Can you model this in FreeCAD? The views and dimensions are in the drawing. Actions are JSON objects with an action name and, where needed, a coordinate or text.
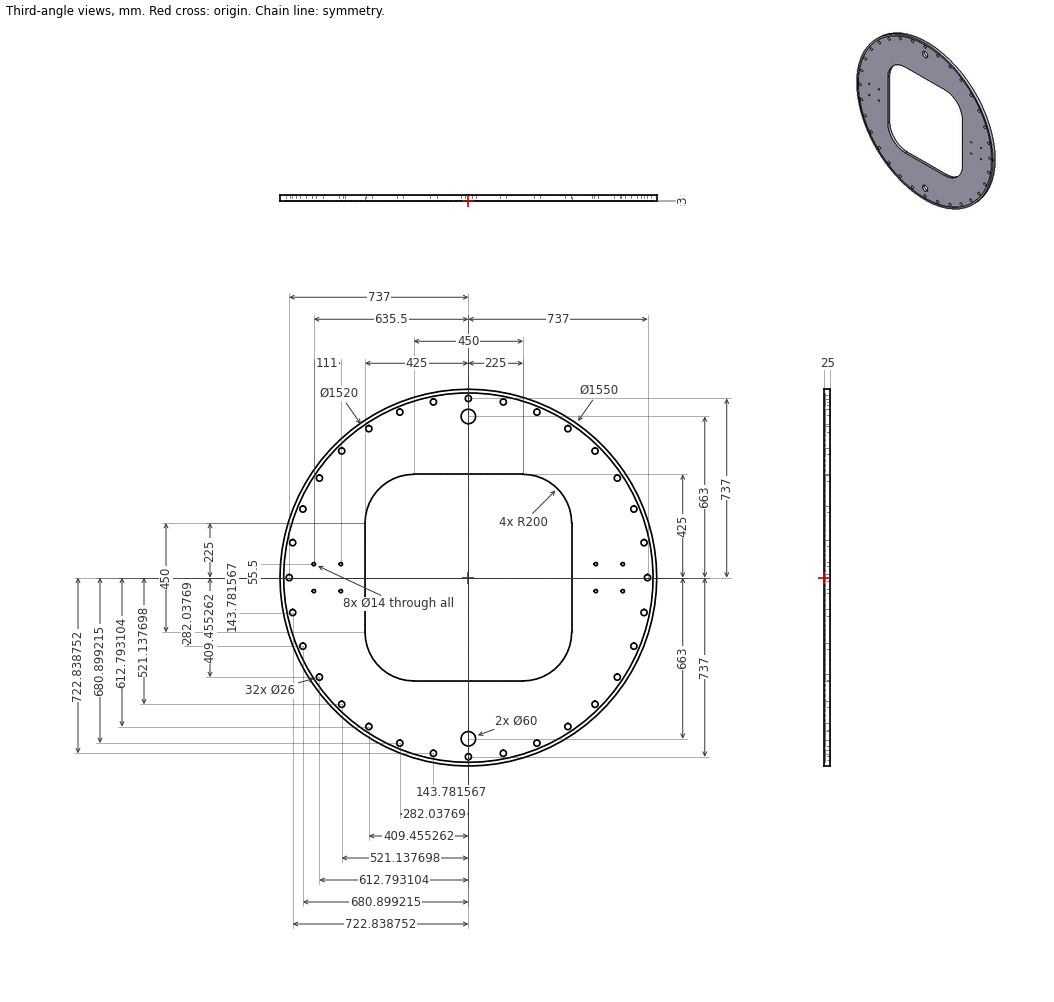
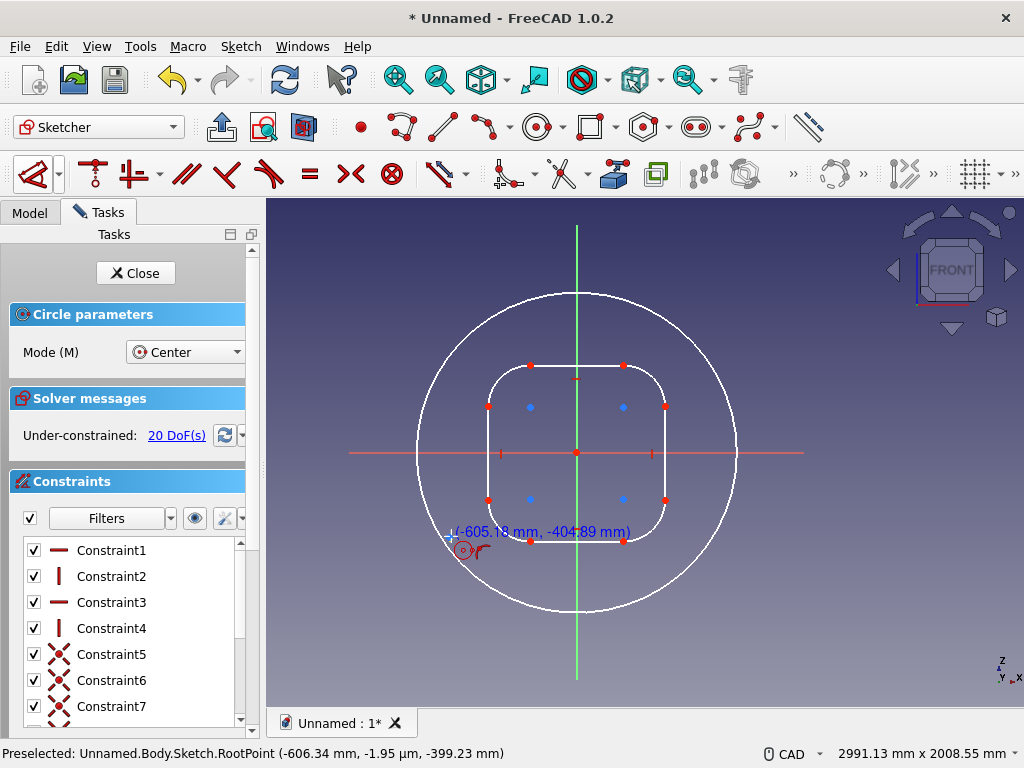
{"action": "scroll", "coordinate": [492, 580], "scroll_direction": "up", "scroll_amount": 11}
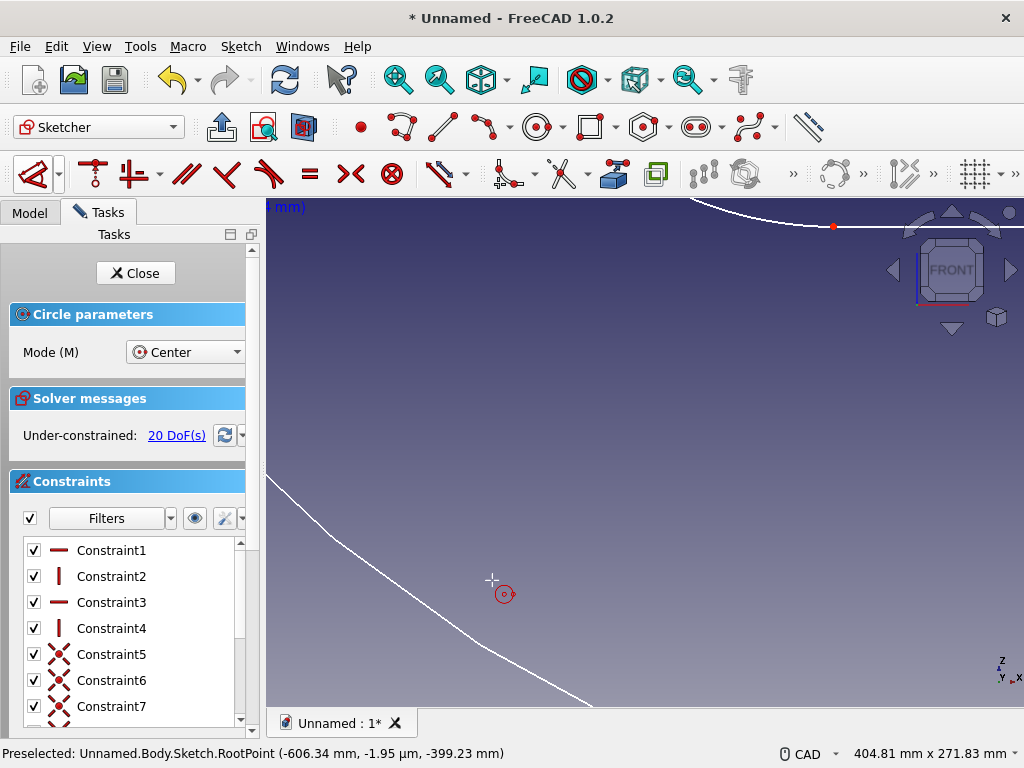
{"action": "scroll", "coordinate": [492, 581], "scroll_direction": "down", "scroll_amount": 11}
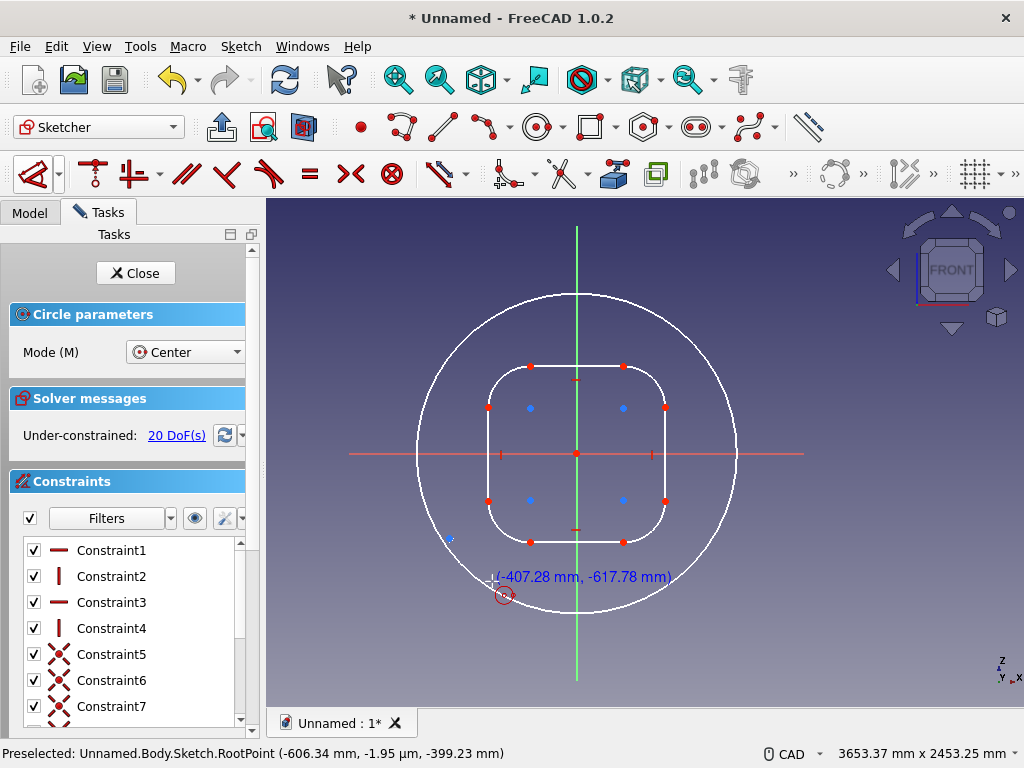
{"action": "scroll", "coordinate": [492, 581], "scroll_direction": "up", "scroll_amount": 4}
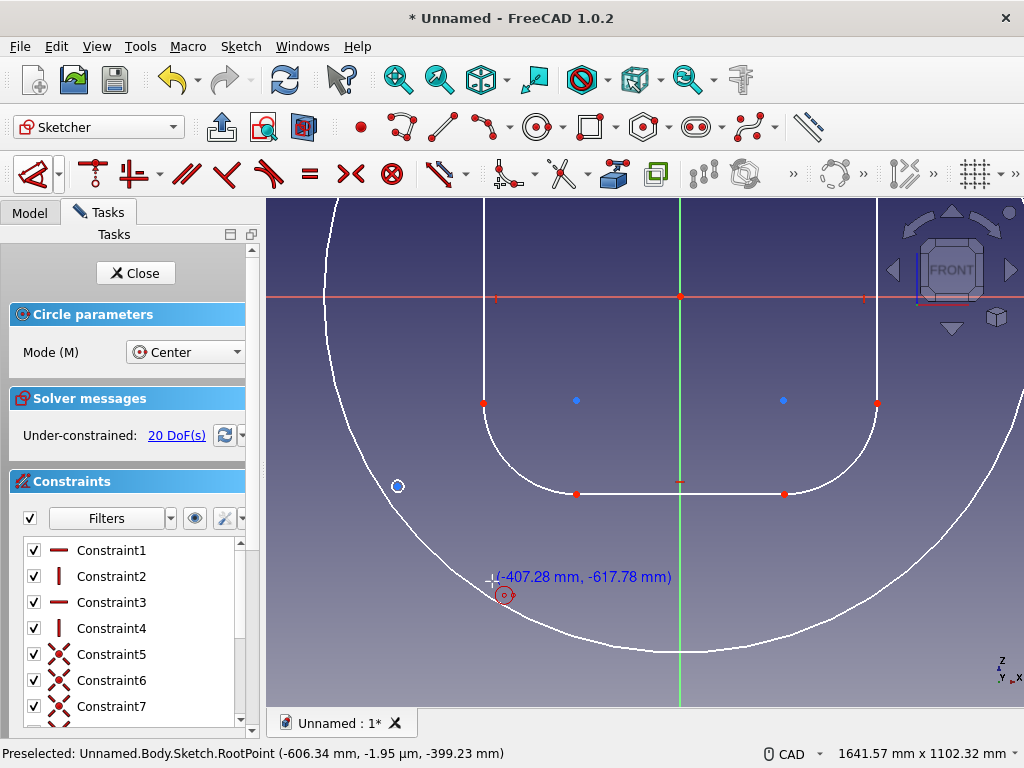
{"action": "left_click", "coordinate": [491, 580]}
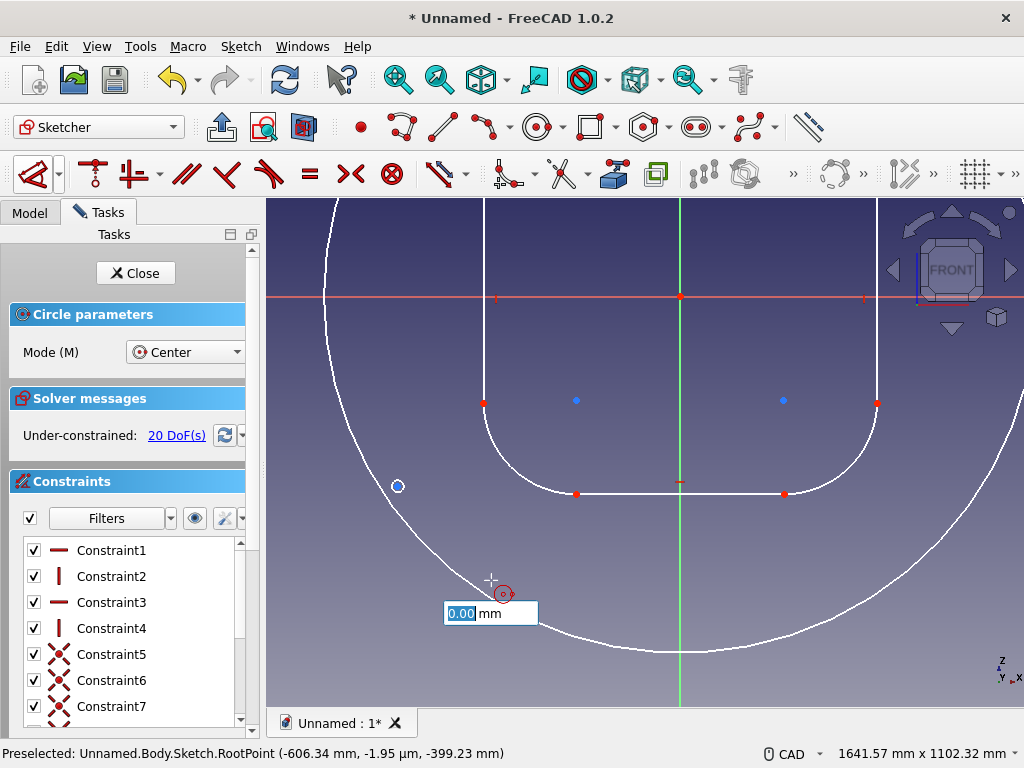
{"action": "scroll", "coordinate": [495, 575], "scroll_direction": "up", "scroll_amount": 5}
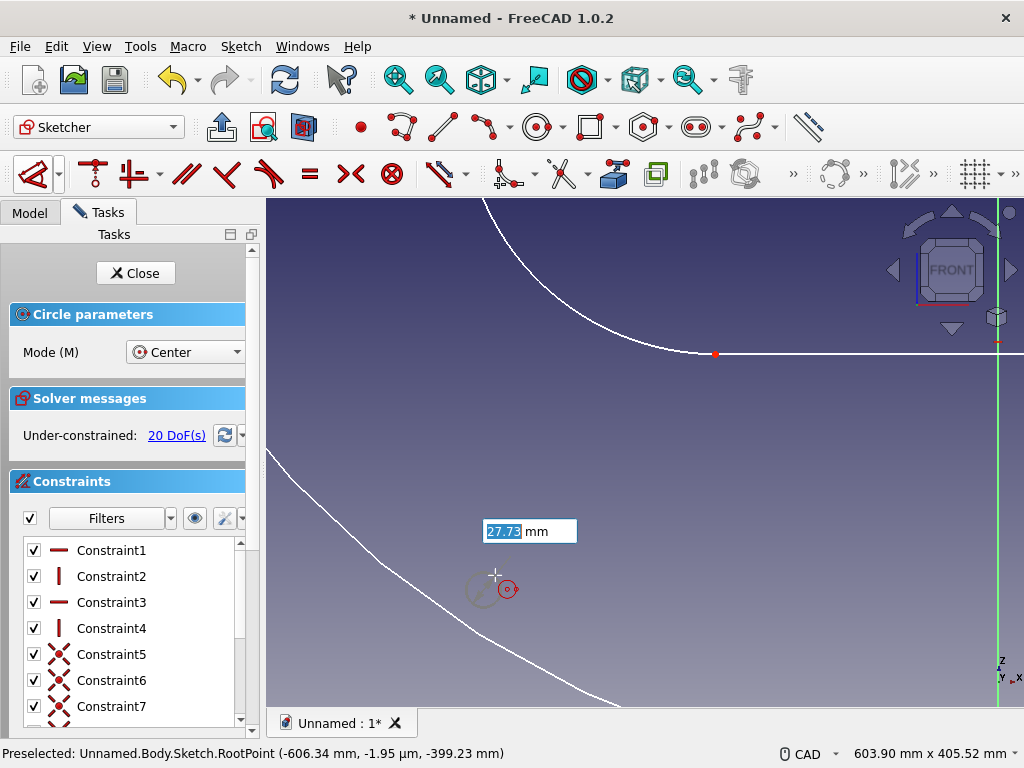
{"action": "left_click", "coordinate": [496, 574]}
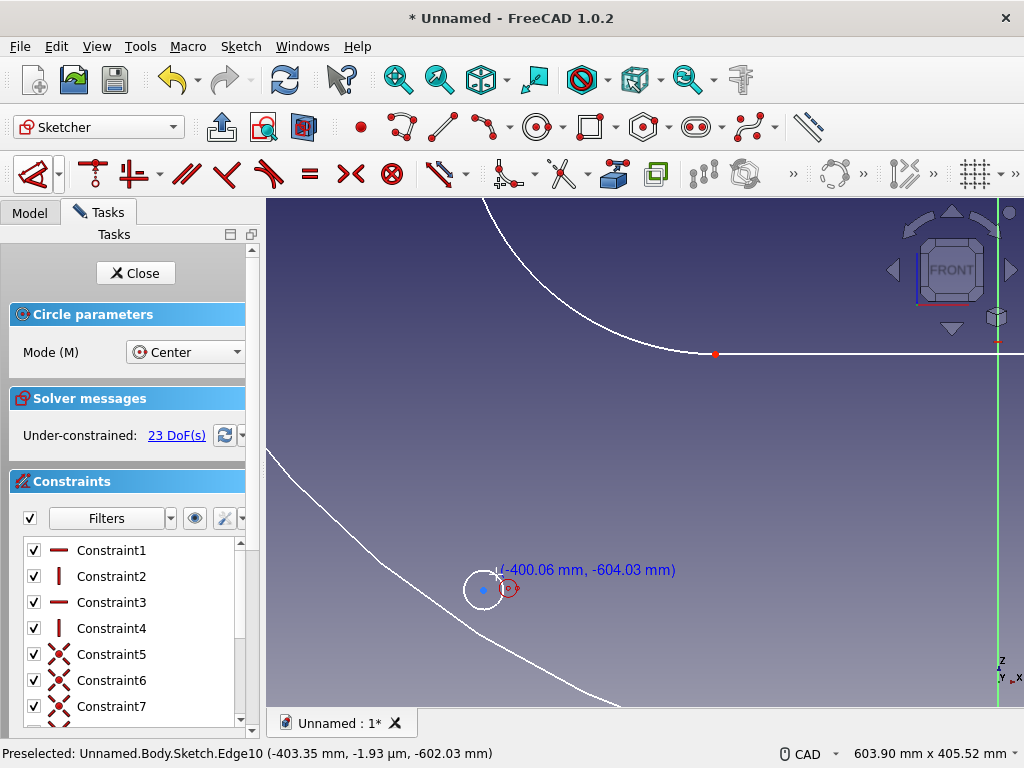
{"action": "scroll", "coordinate": [344, 471], "scroll_direction": "up", "scroll_amount": 2}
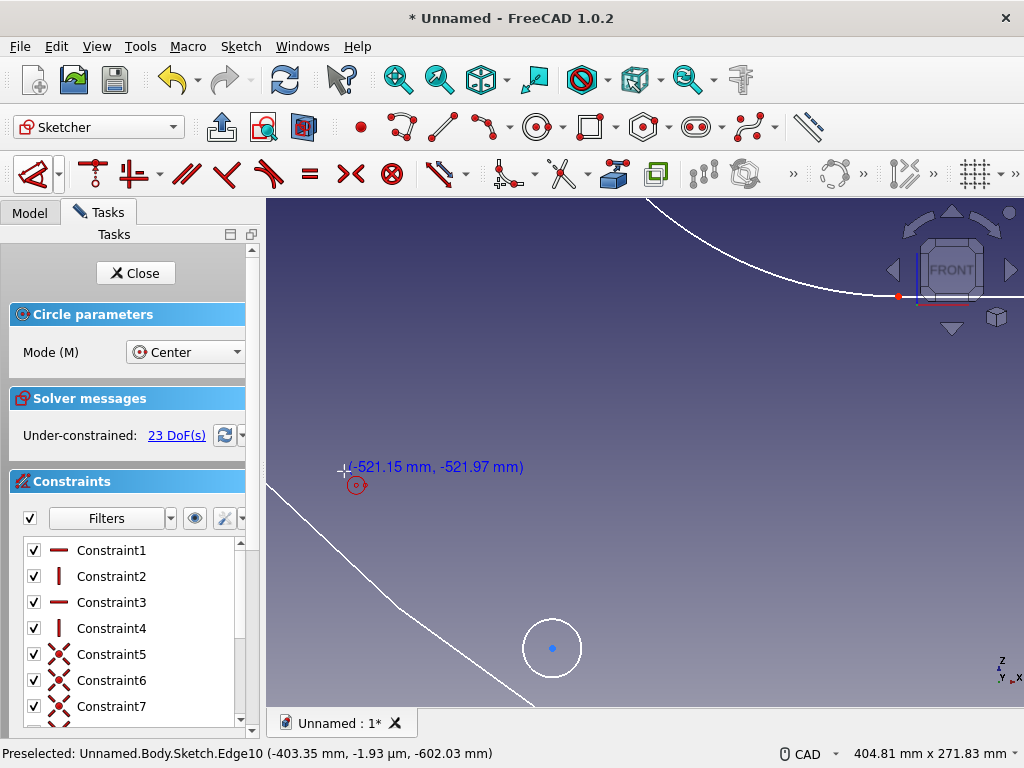
{"action": "scroll", "coordinate": [484, 572], "scroll_direction": "down", "scroll_amount": 11}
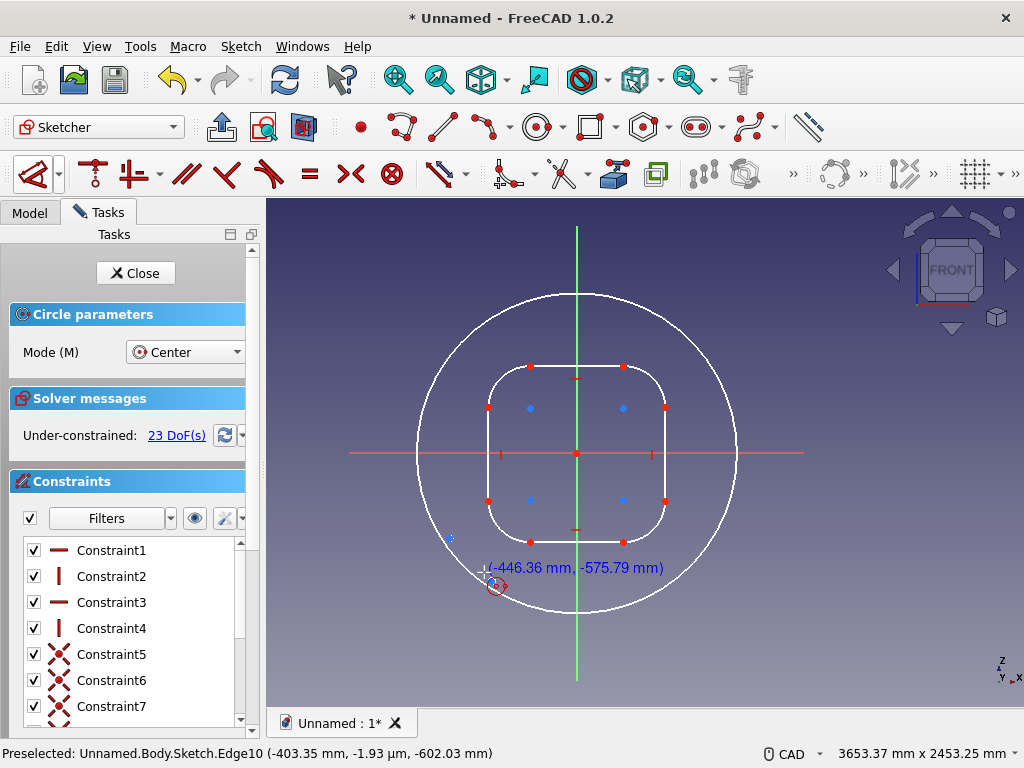
{"action": "scroll", "coordinate": [469, 561], "scroll_direction": "up", "scroll_amount": 4}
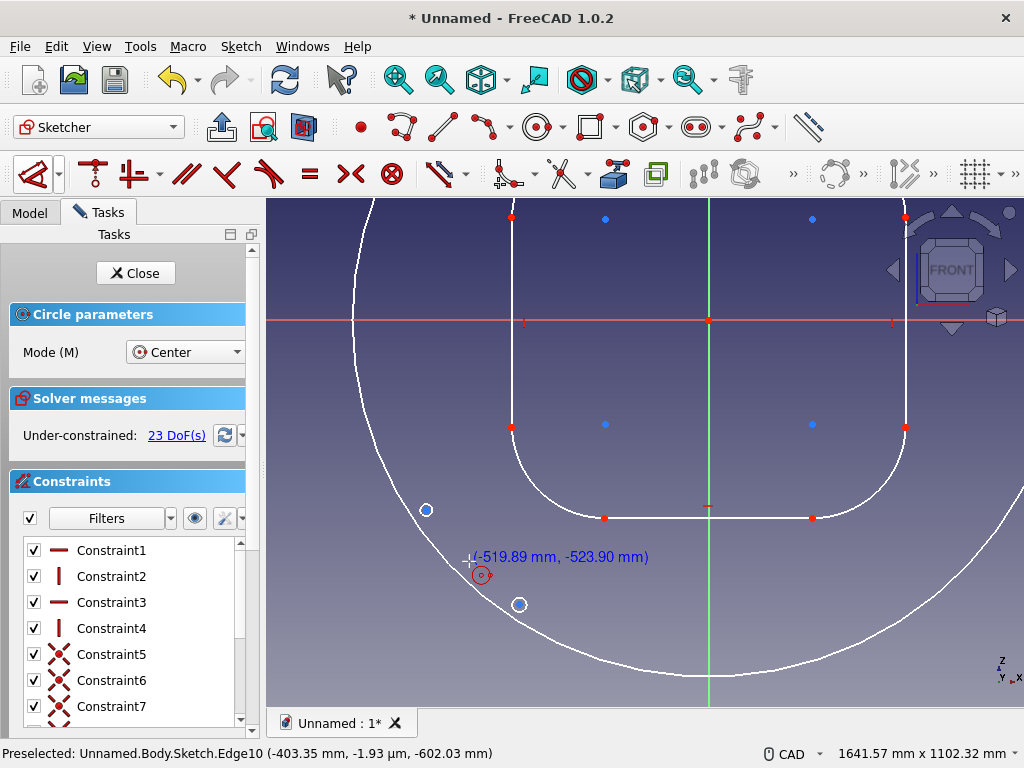
{"action": "left_click", "coordinate": [468, 561]}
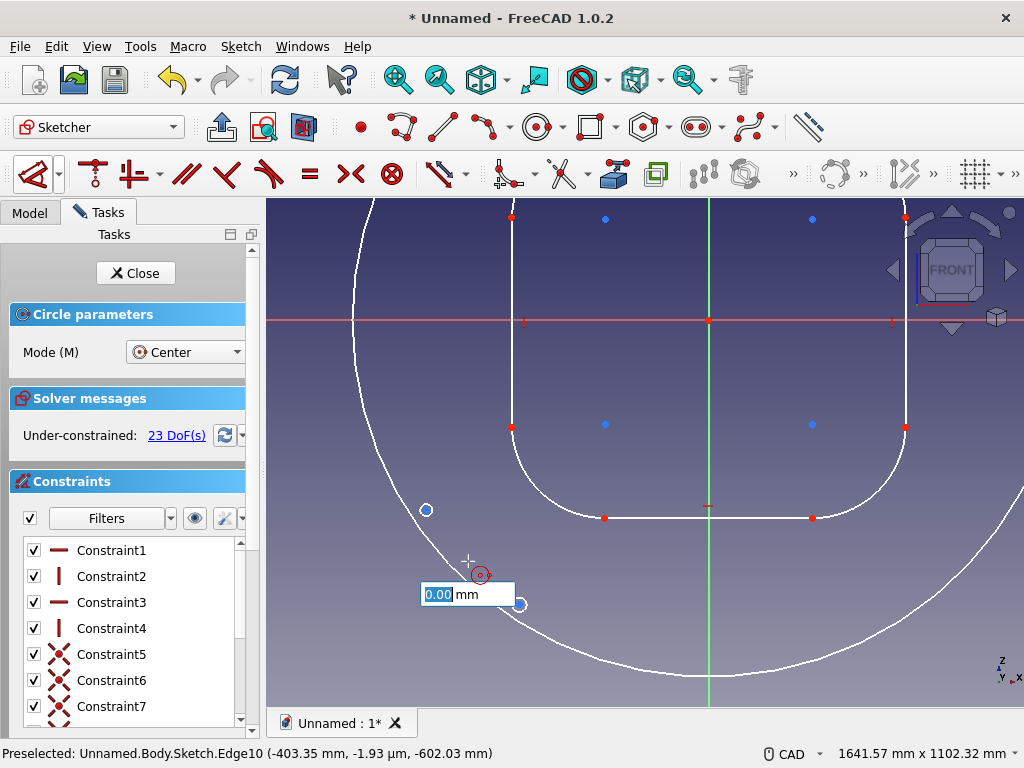
{"action": "scroll", "coordinate": [472, 557], "scroll_direction": "up", "scroll_amount": 5}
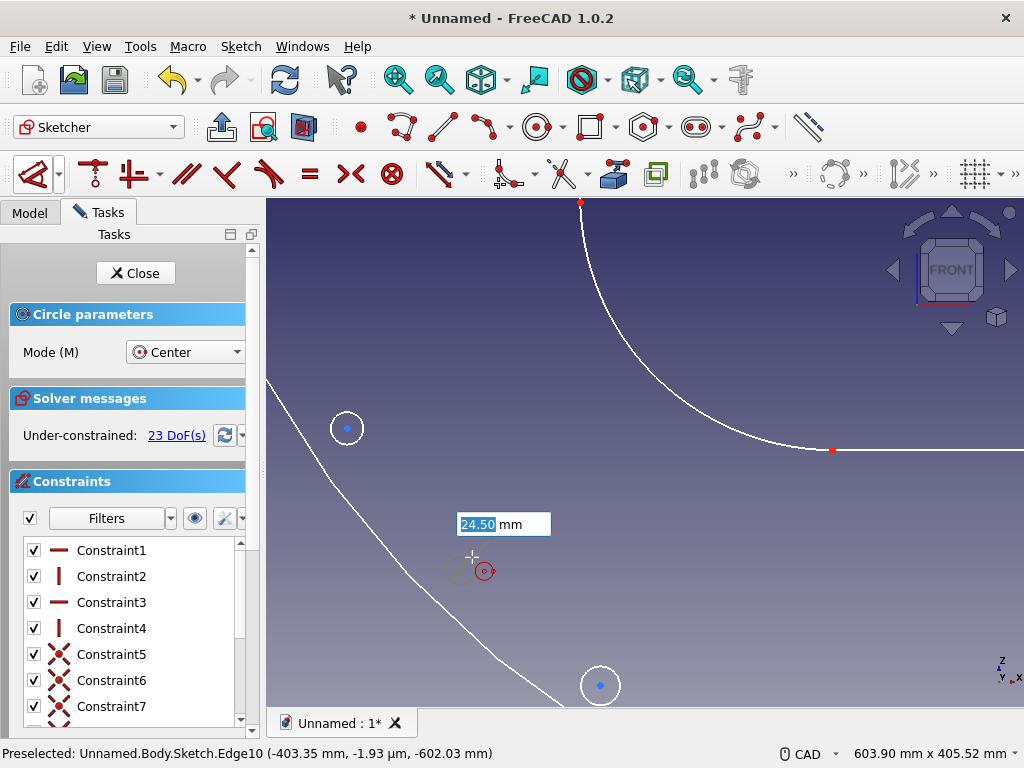
{"action": "left_click", "coordinate": [472, 555]}